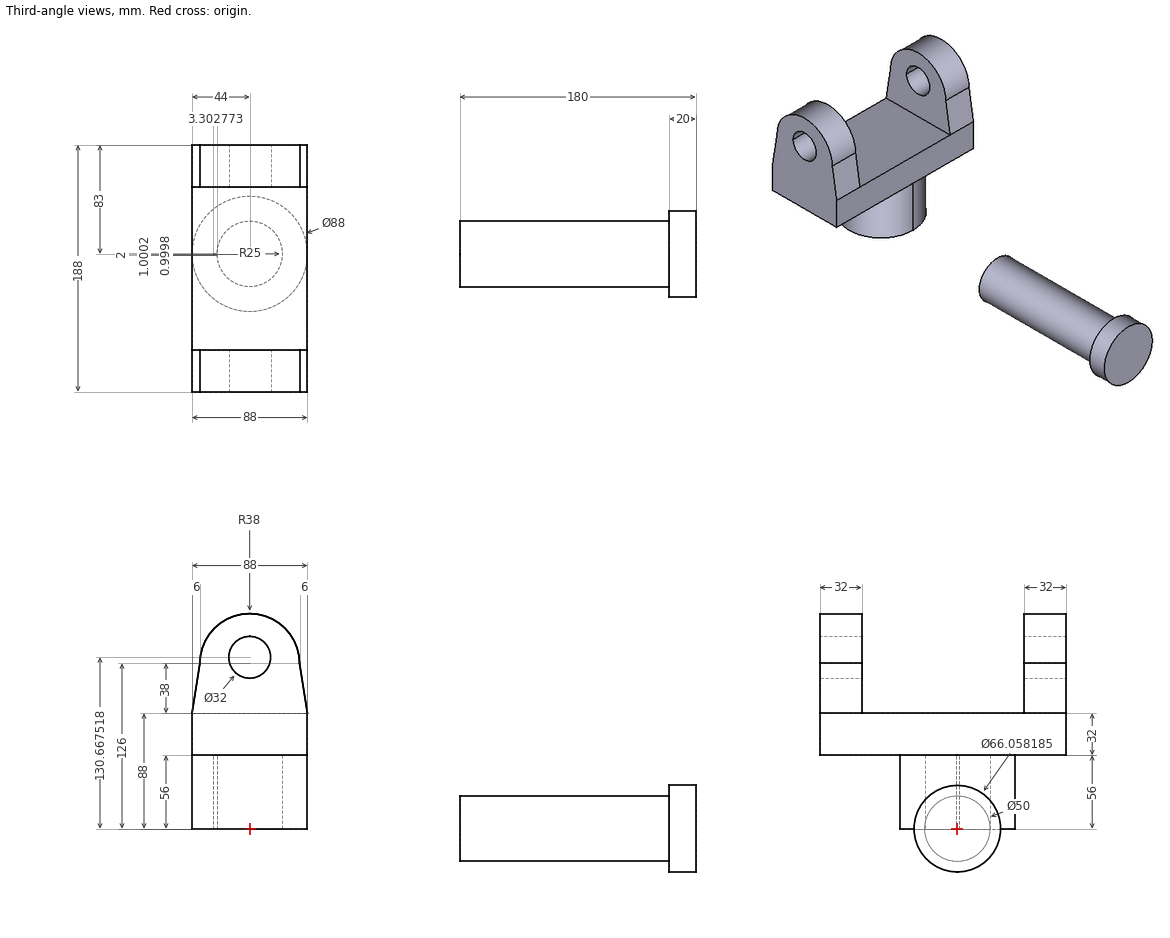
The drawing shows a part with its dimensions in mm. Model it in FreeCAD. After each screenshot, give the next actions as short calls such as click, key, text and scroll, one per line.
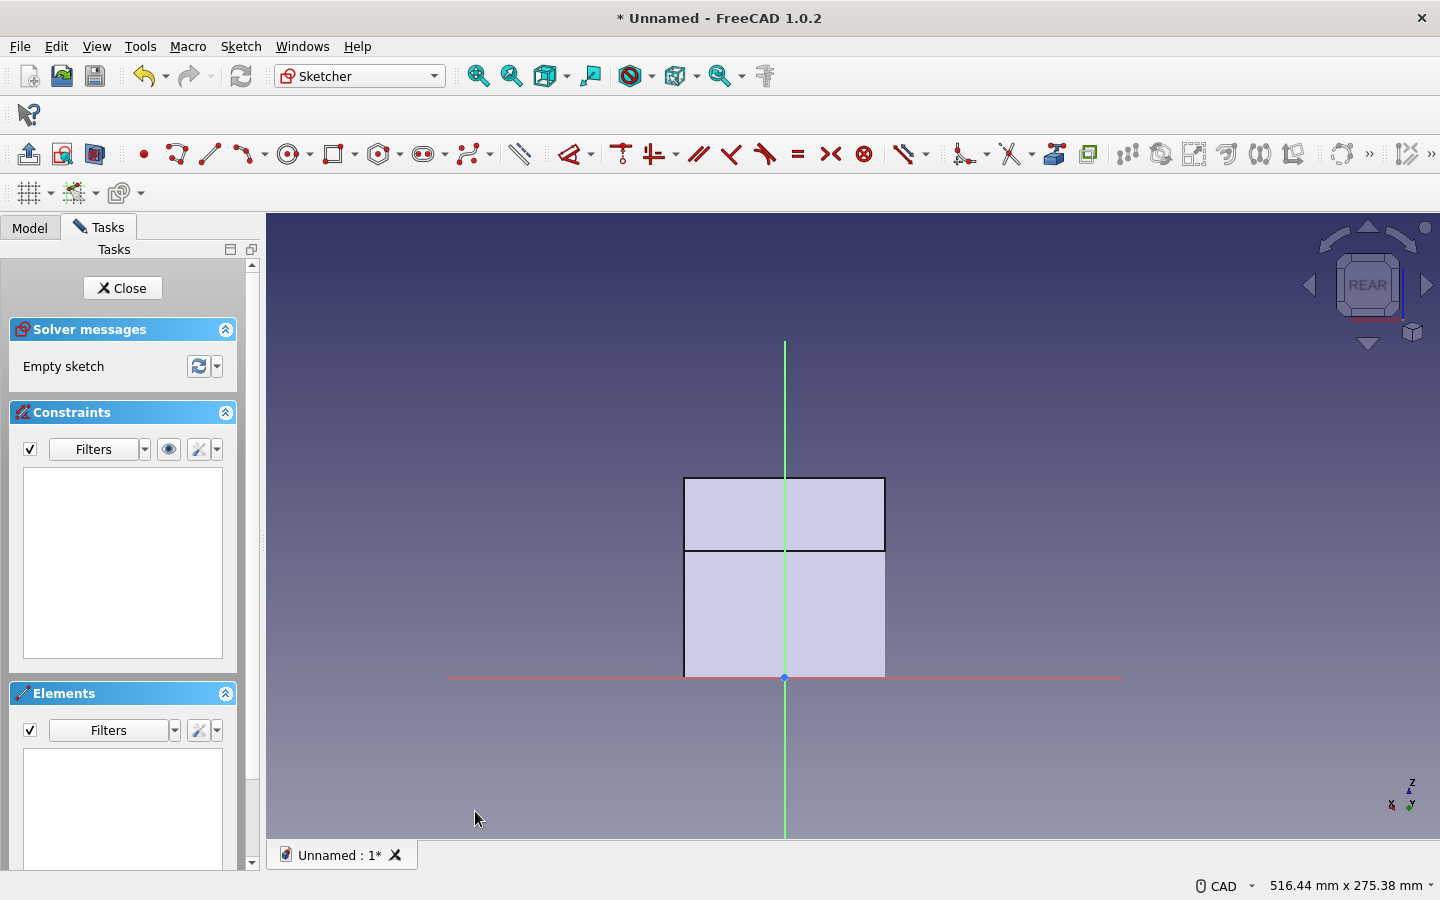
key(g)
key(m)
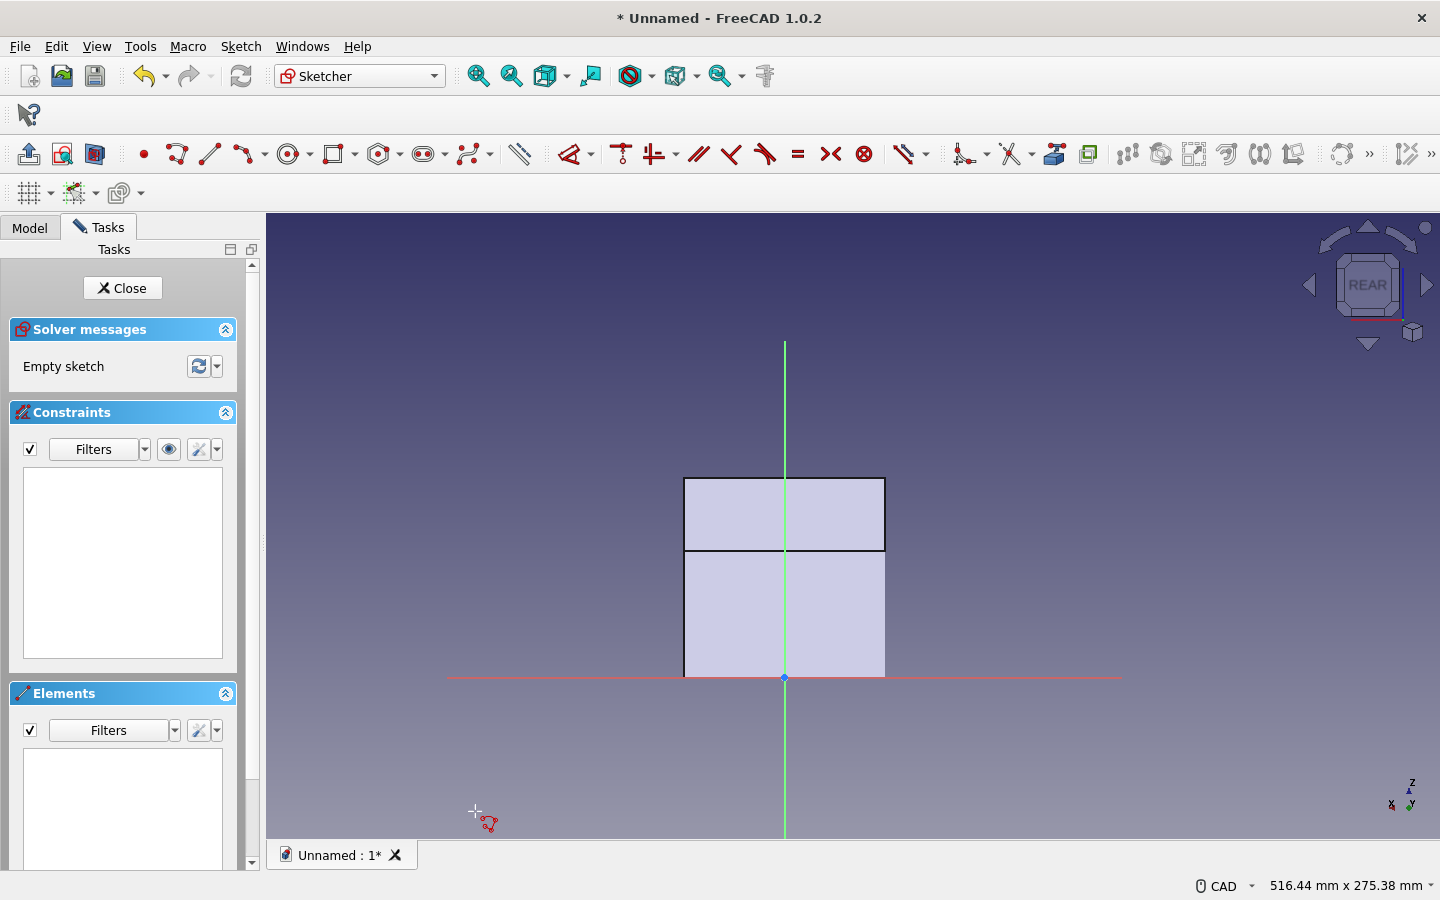
click(698, 391)
click(684, 478)
click(885, 478)
click(871, 391)
right_click(871, 391)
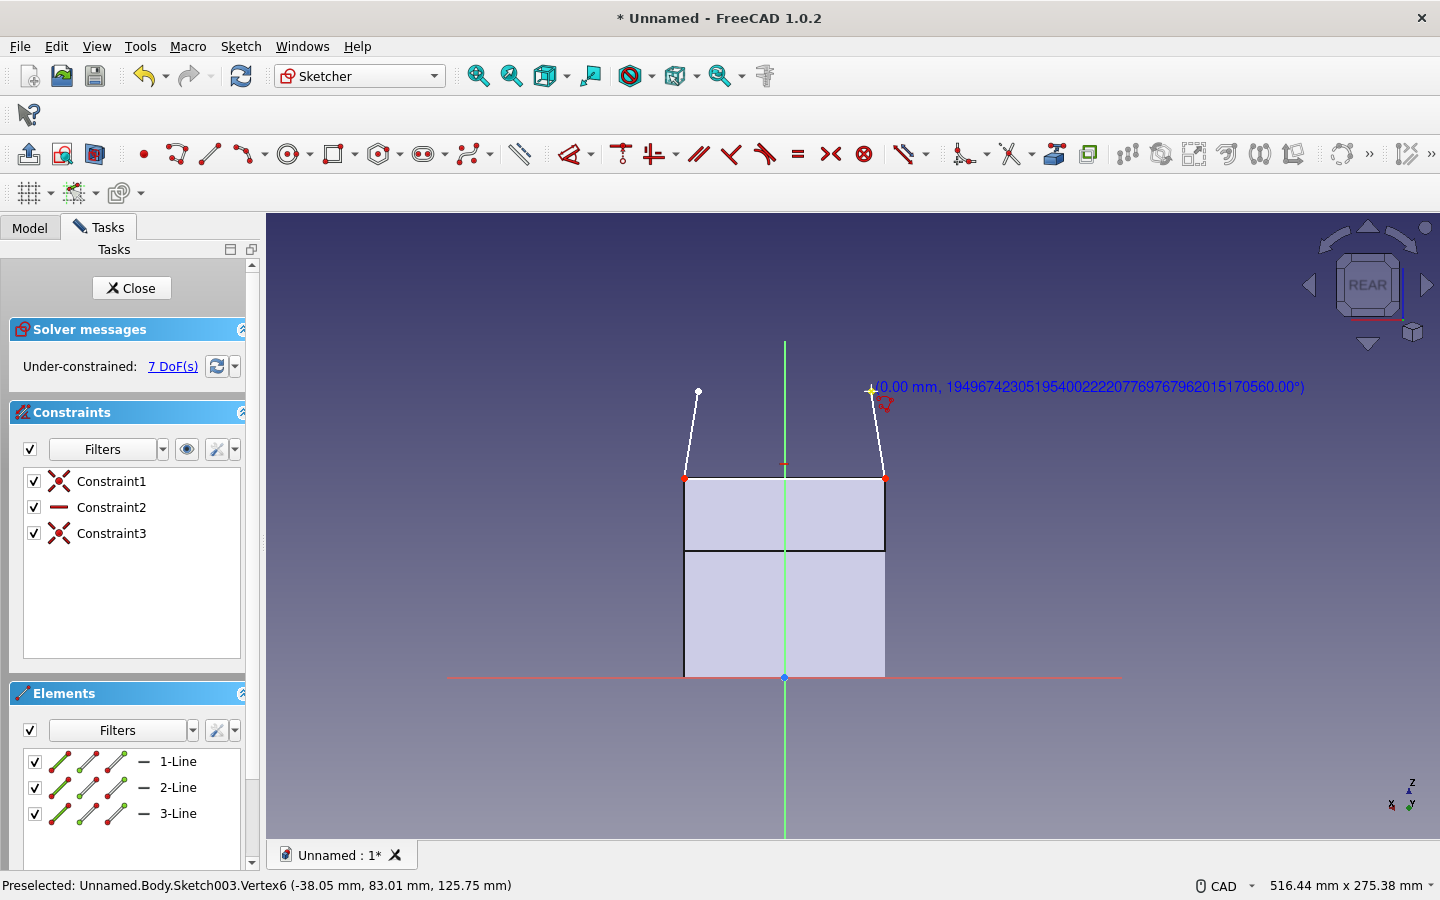
key(g)
key(3)
key(a)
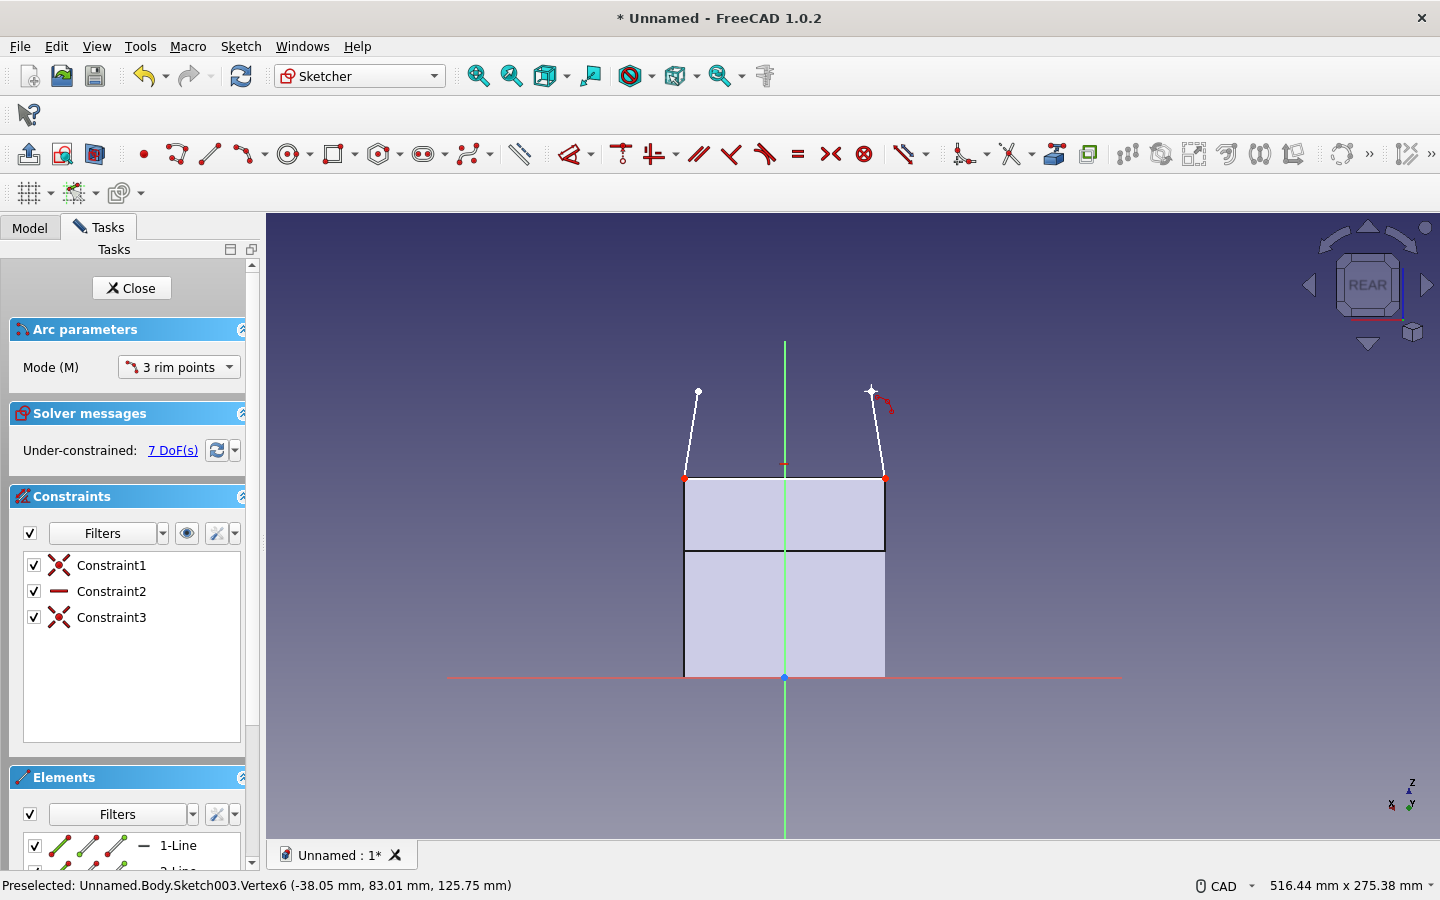
click(871, 392)
click(698, 392)
click(811, 309)
key(Escape)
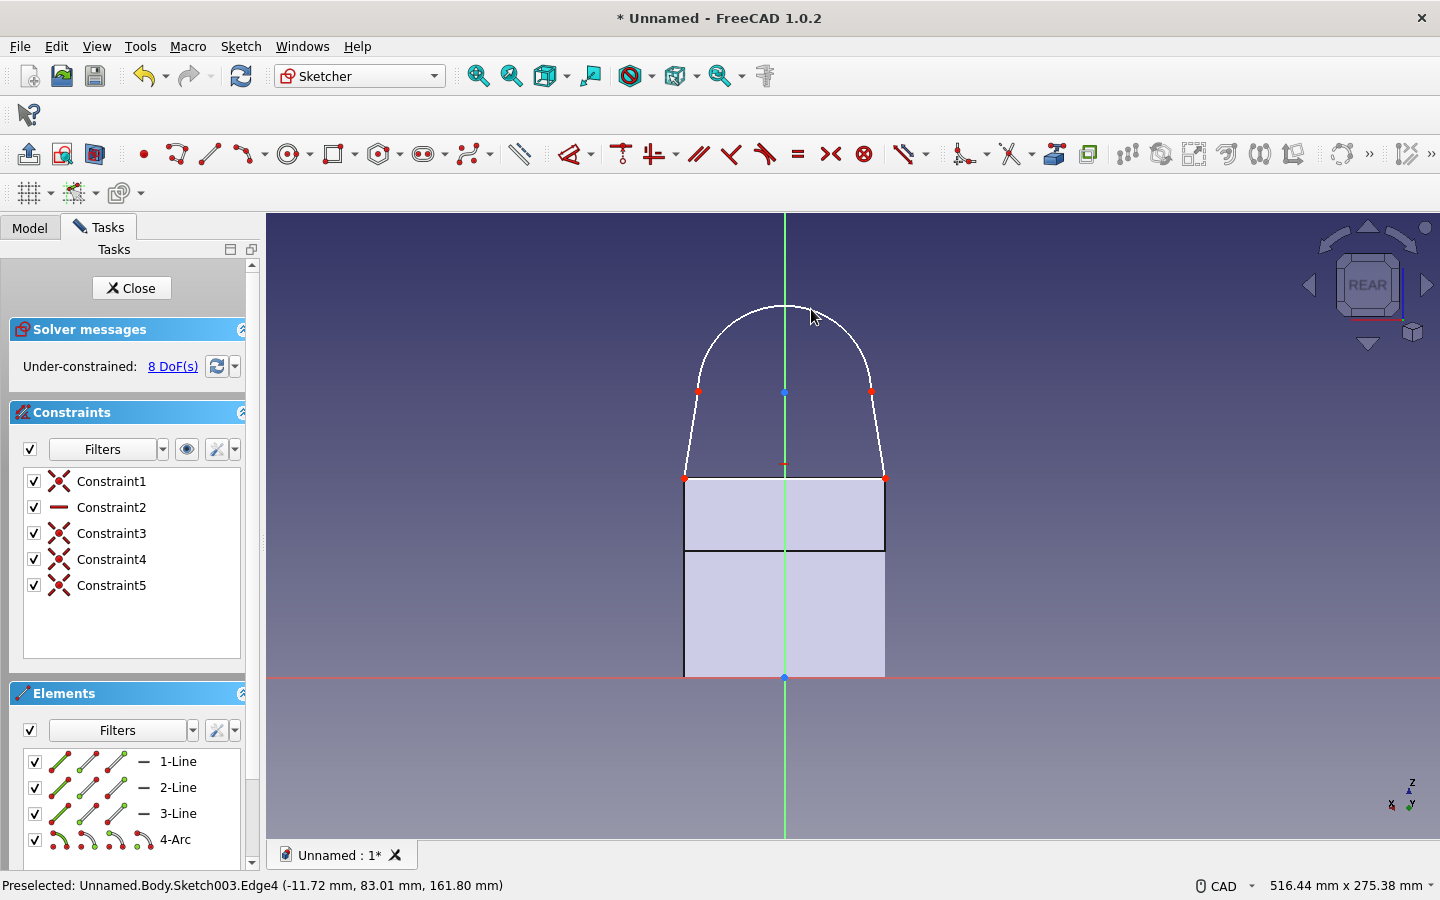
click(785, 392)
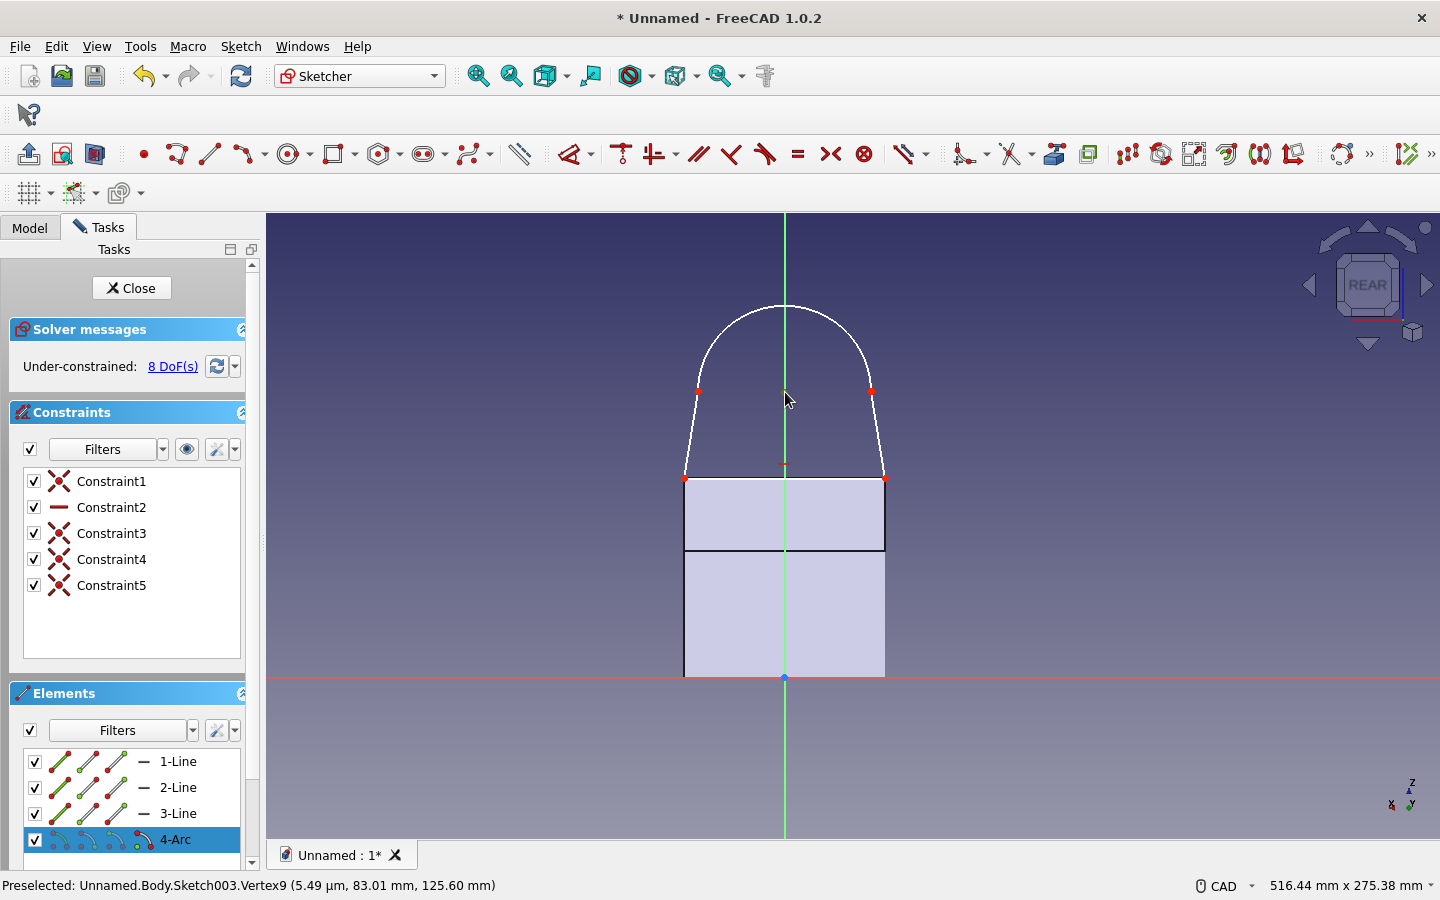
click(785, 770)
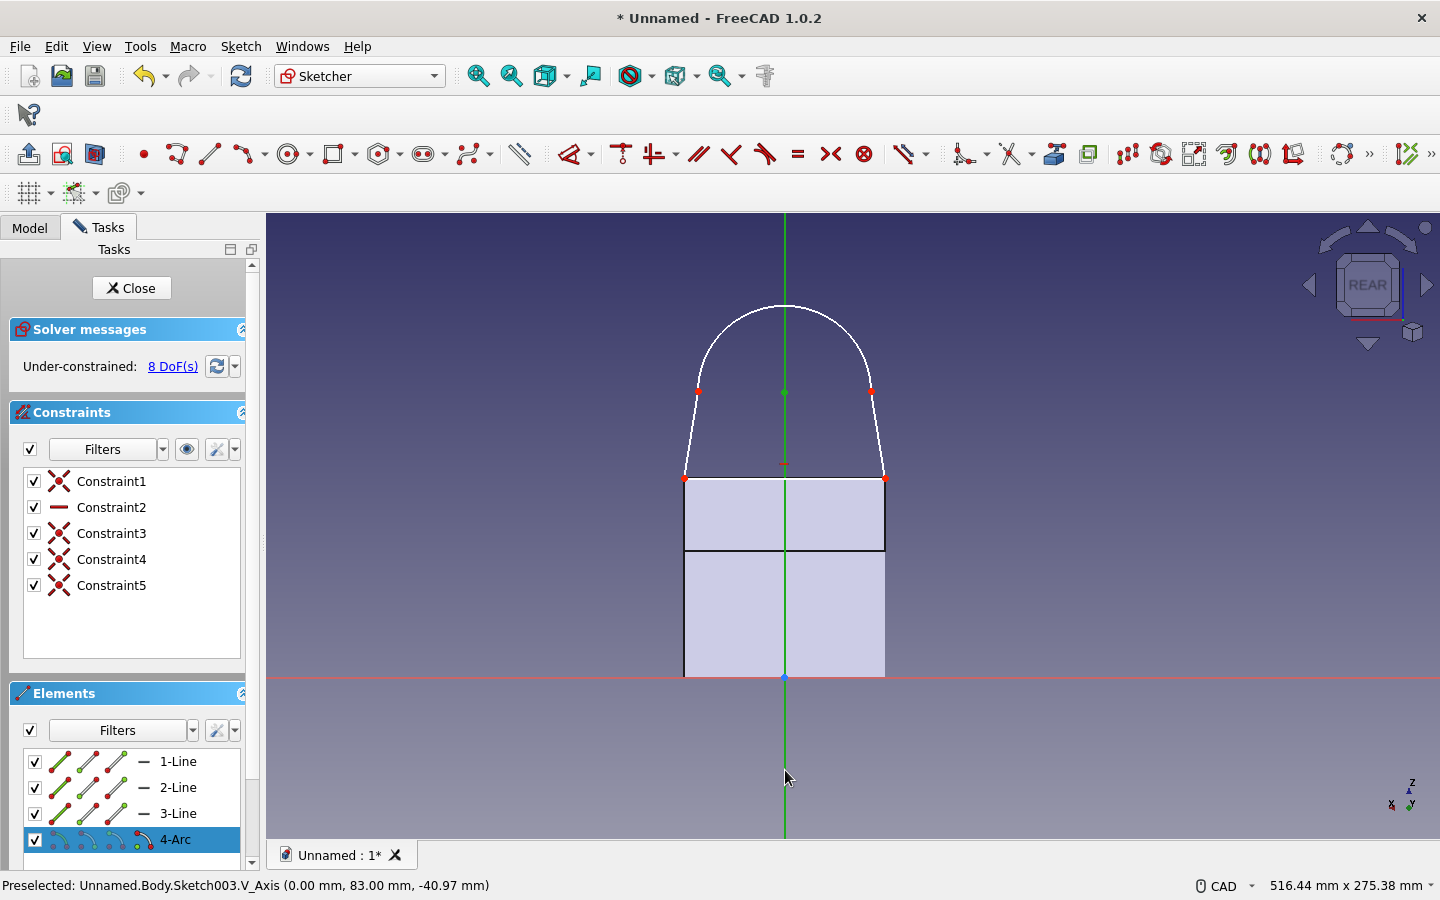
click(621, 154)